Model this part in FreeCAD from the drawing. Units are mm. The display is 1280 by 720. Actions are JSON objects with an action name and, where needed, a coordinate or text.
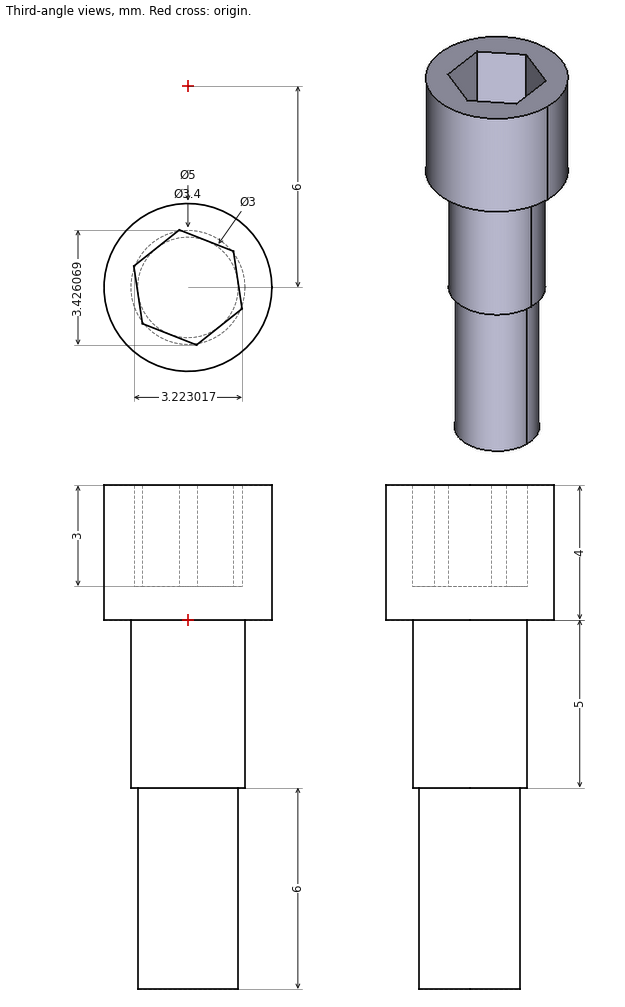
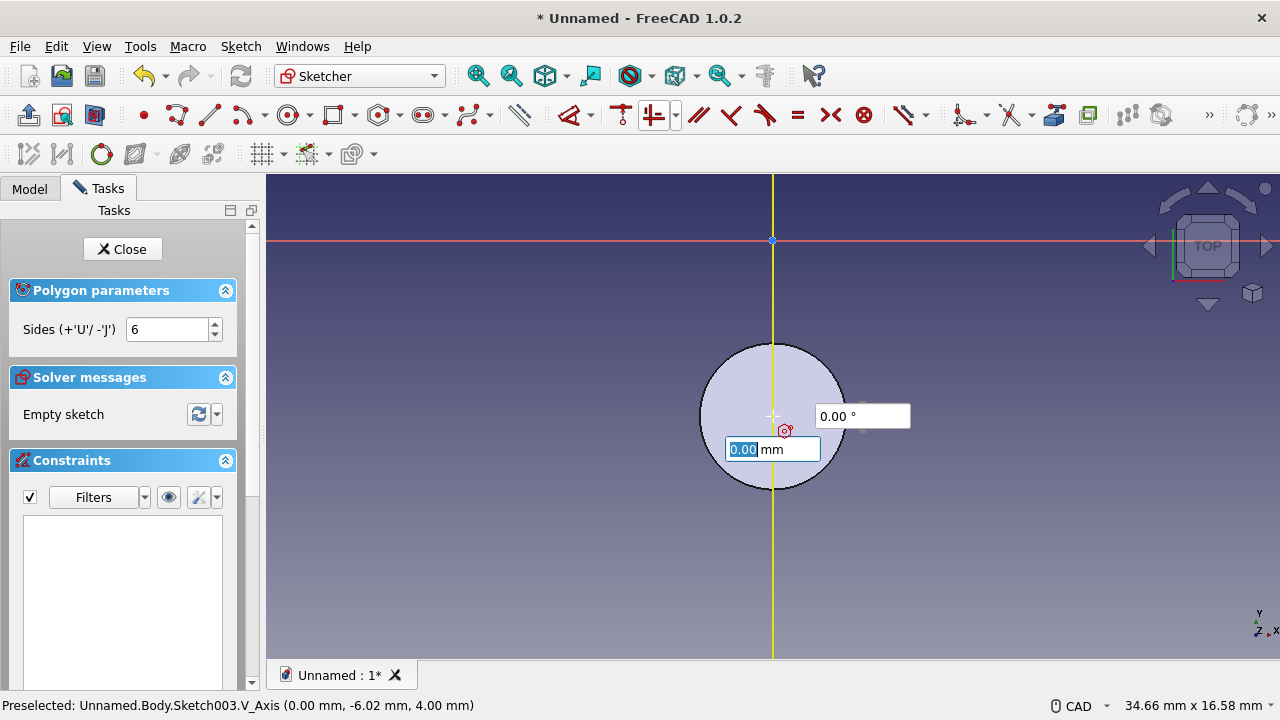
{"action": "left_click", "coordinate": [726, 398]}
{"action": "right_click", "coordinate": [726, 398]}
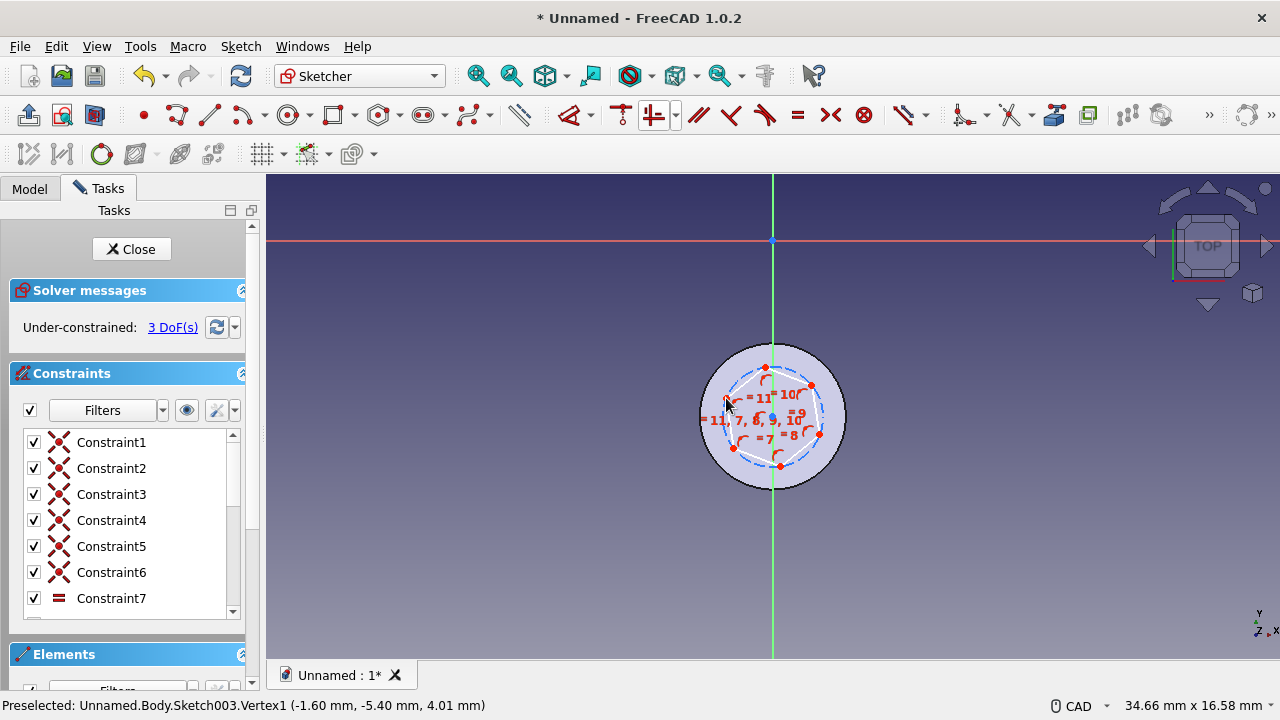
{"action": "key", "text": "d"}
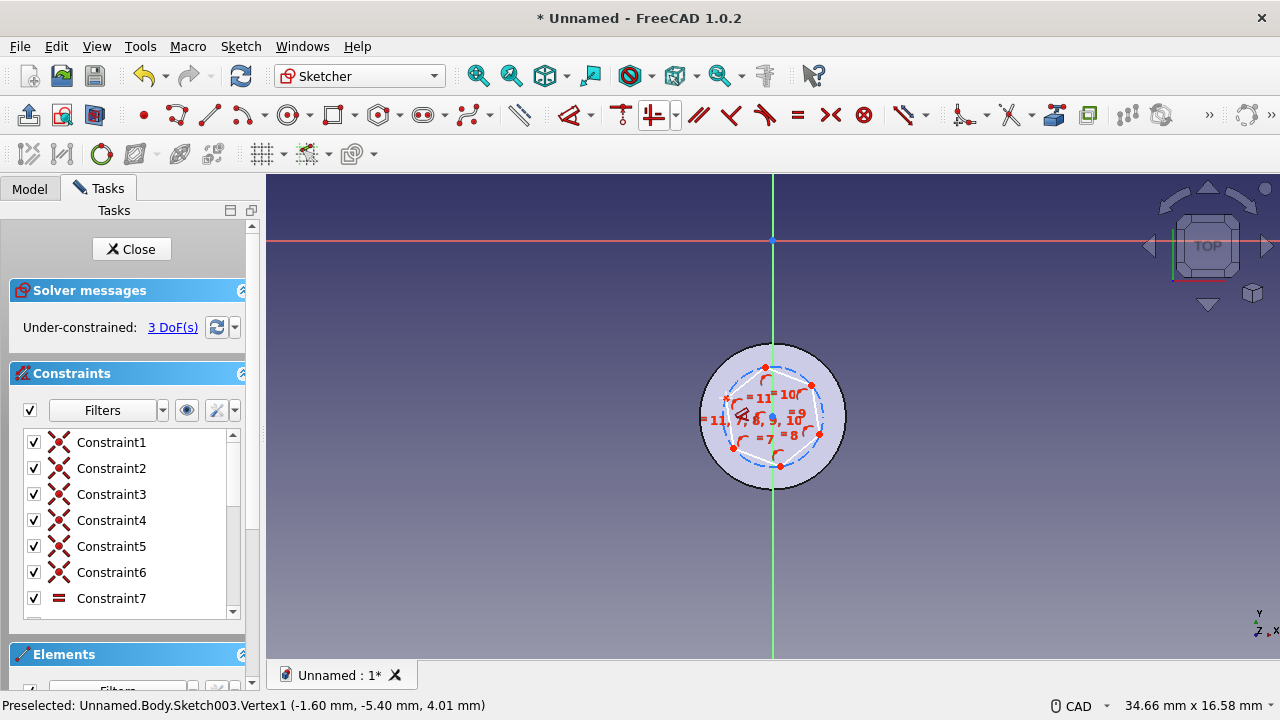
{"action": "left_click", "coordinate": [773, 417]}
{"action": "left_click", "coordinate": [807, 329]}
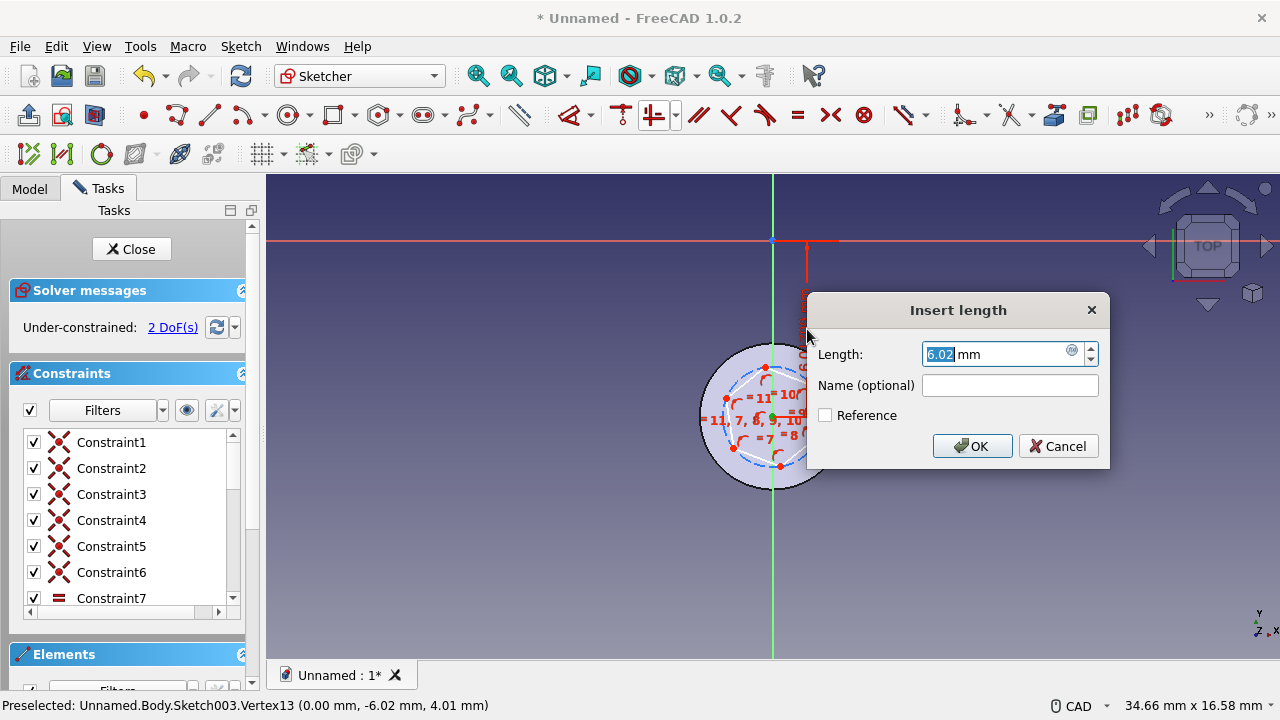
{"action": "type", "text": "6"}
{"action": "key", "text": "Return"}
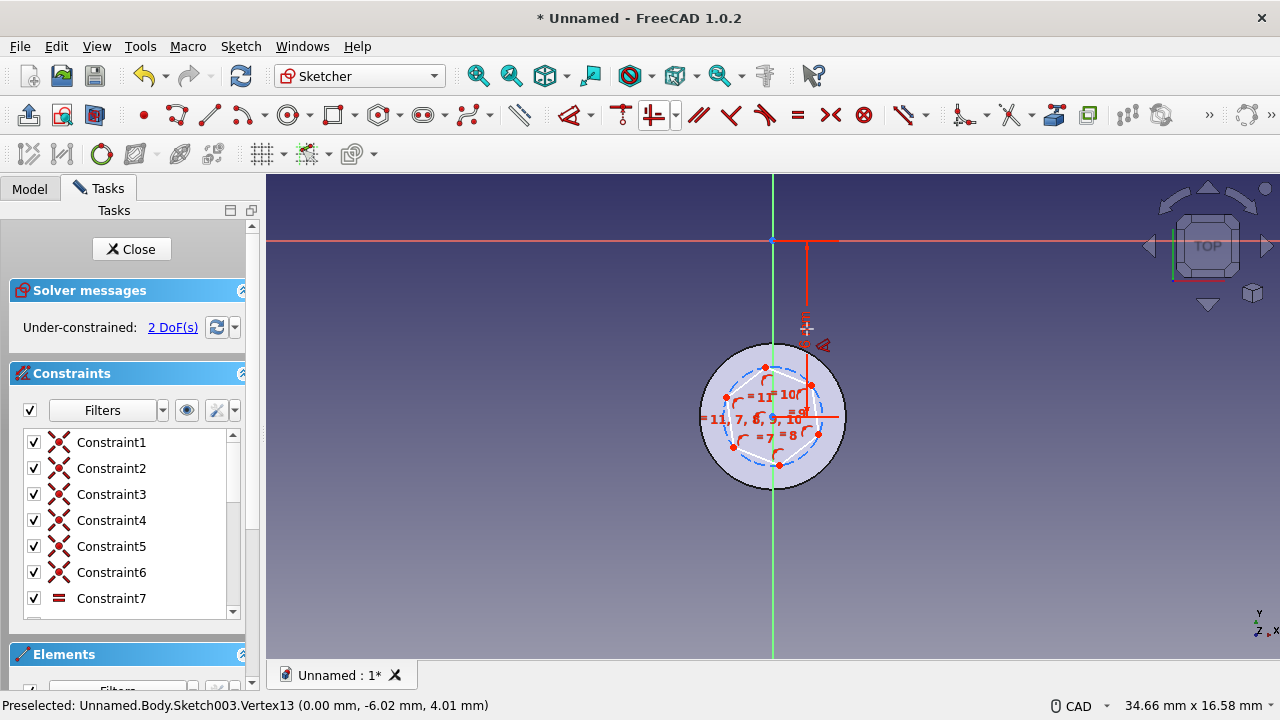
{"action": "left_click", "coordinate": [727, 398]}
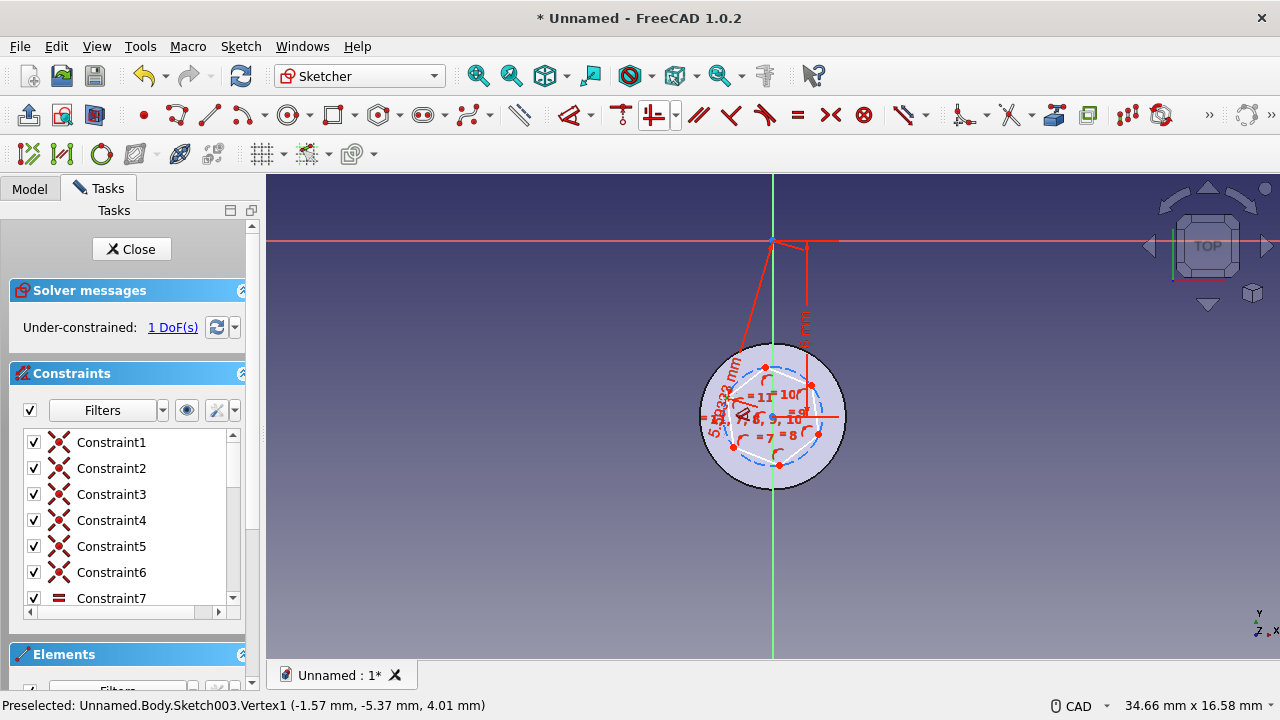
{"action": "left_click", "coordinate": [819, 435]}
{"action": "left_click", "coordinate": [752, 493]}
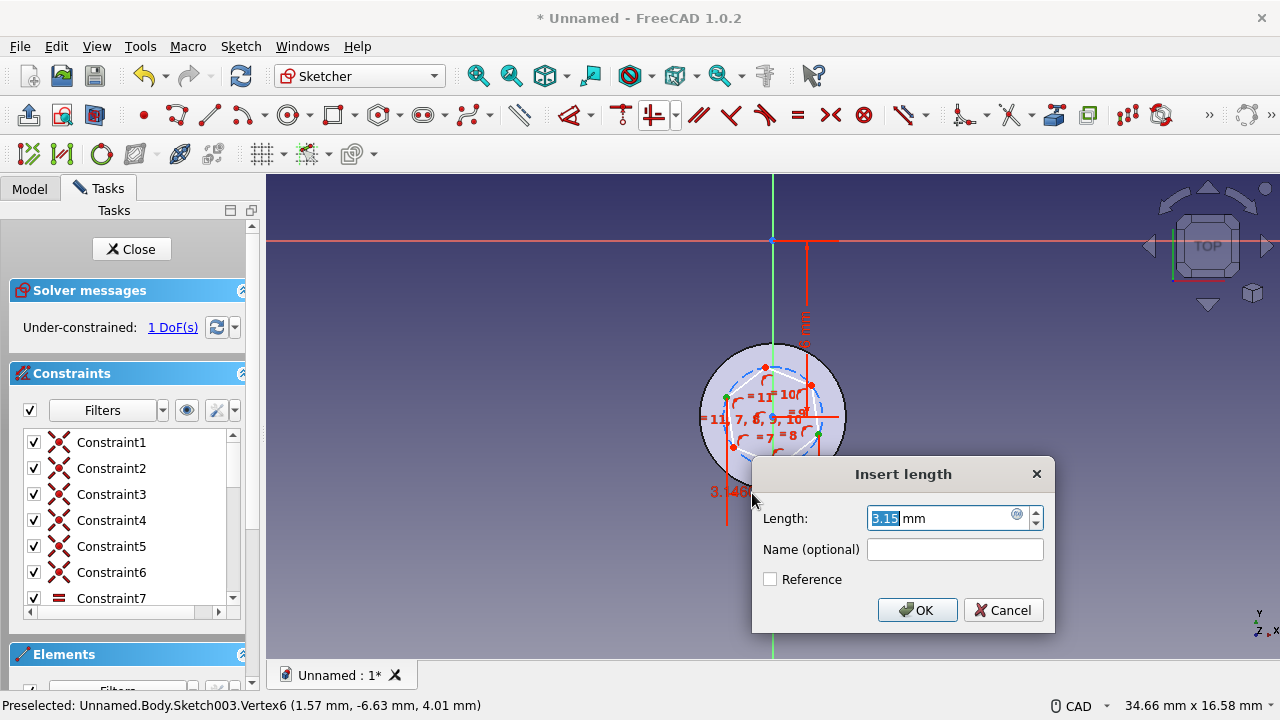
{"action": "type", "text": "3.223017"}
{"action": "key", "text": "Return"}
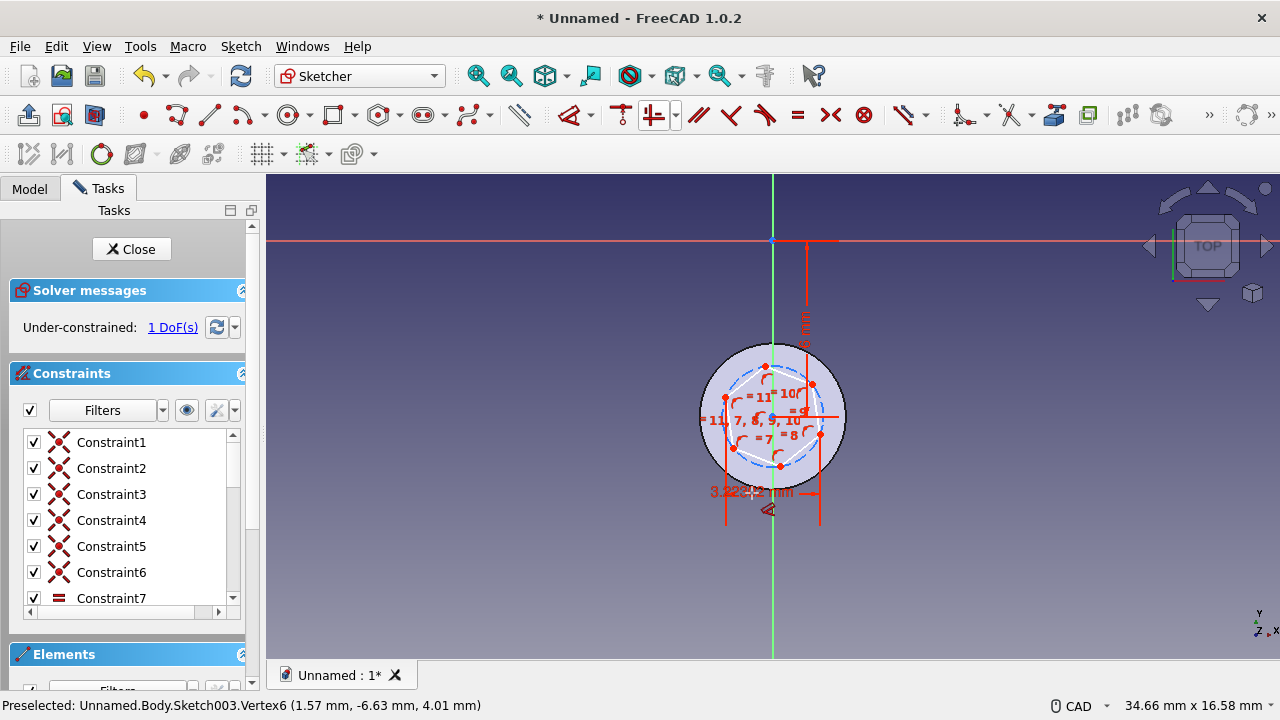
{"action": "left_click", "coordinate": [780, 467]}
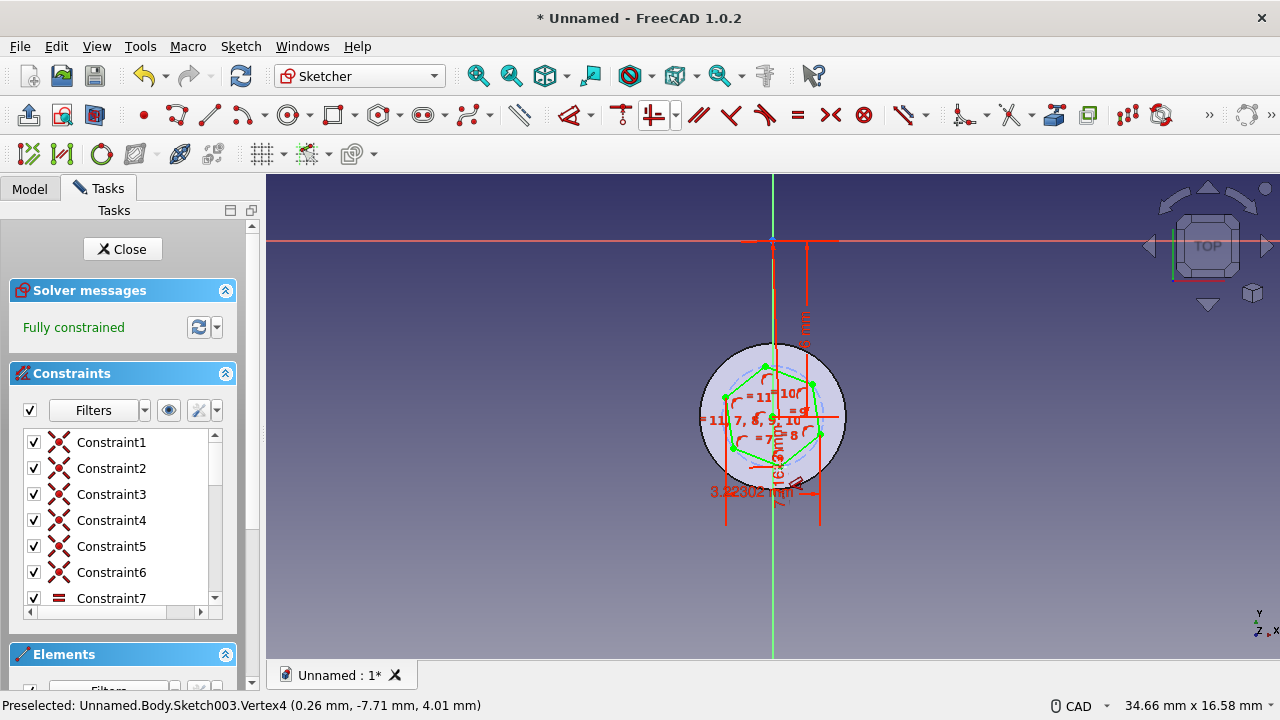
{"action": "left_click", "coordinate": [765, 366]}
{"action": "left_click", "coordinate": [838, 416]}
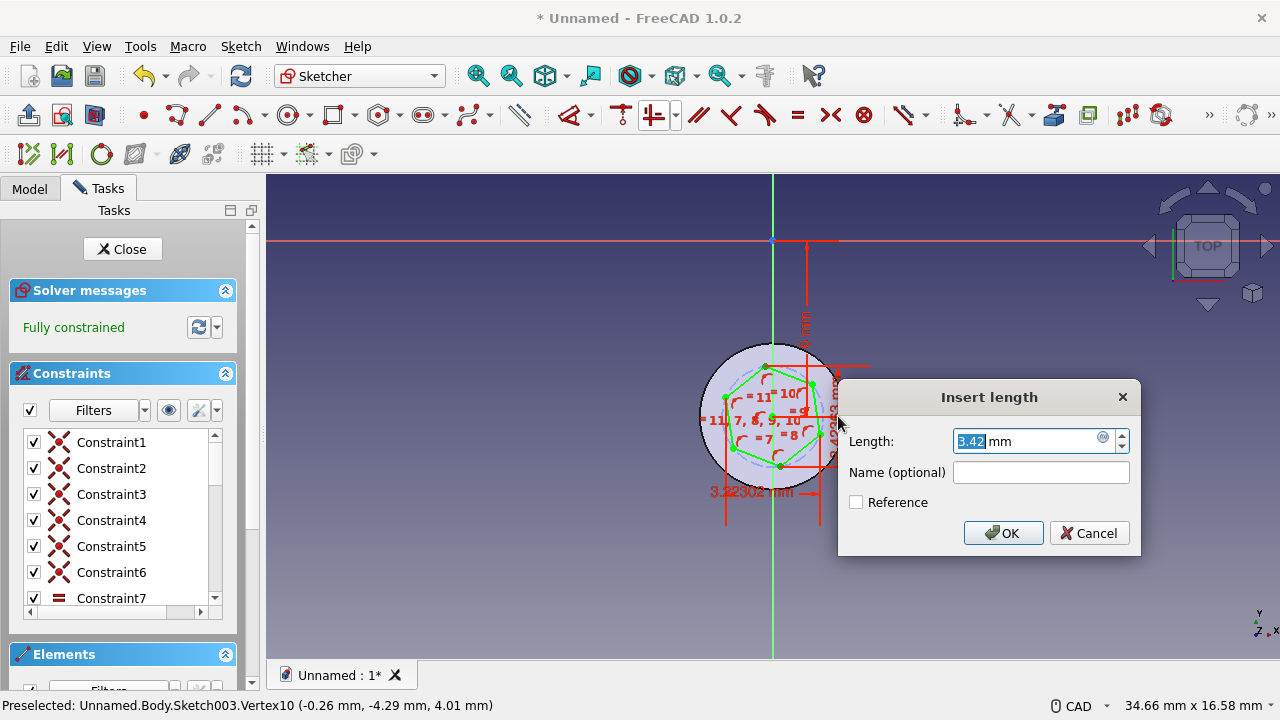
{"action": "type", "text": "3.426069"}
{"action": "key", "text": "Return"}
{"action": "key", "text": "Escape"}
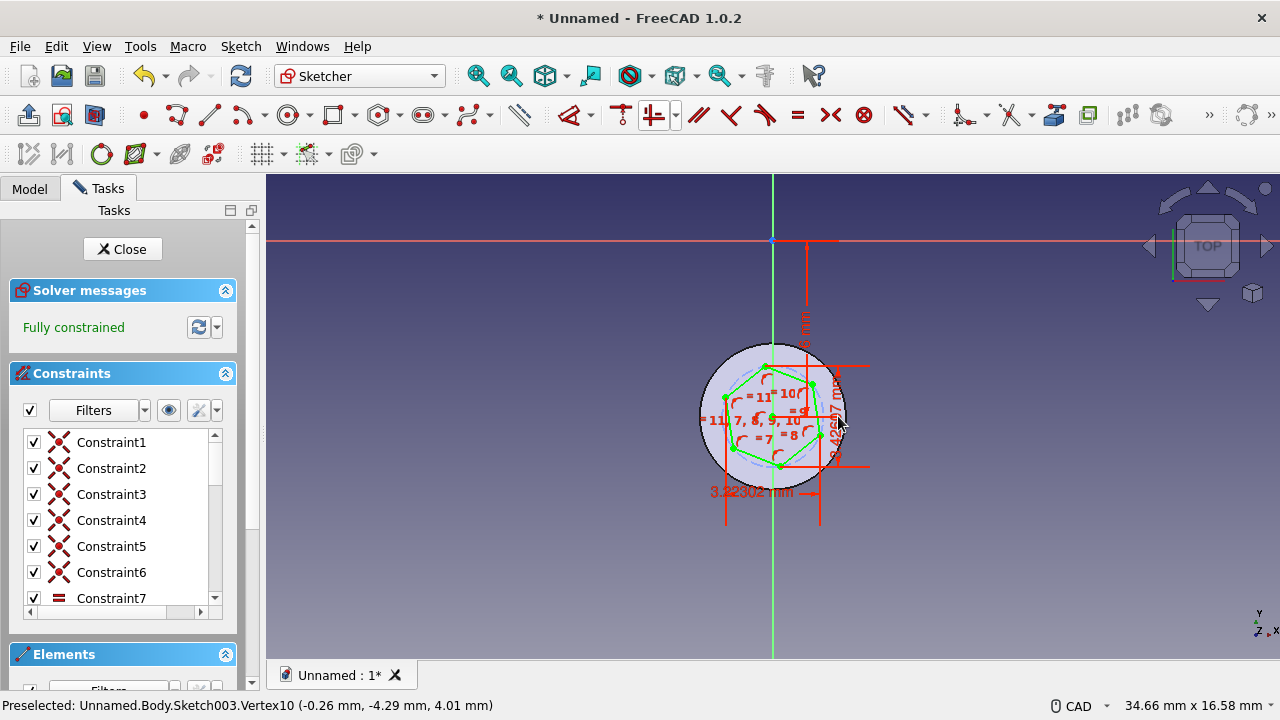
{"action": "left_click", "coordinate": [123, 249]}